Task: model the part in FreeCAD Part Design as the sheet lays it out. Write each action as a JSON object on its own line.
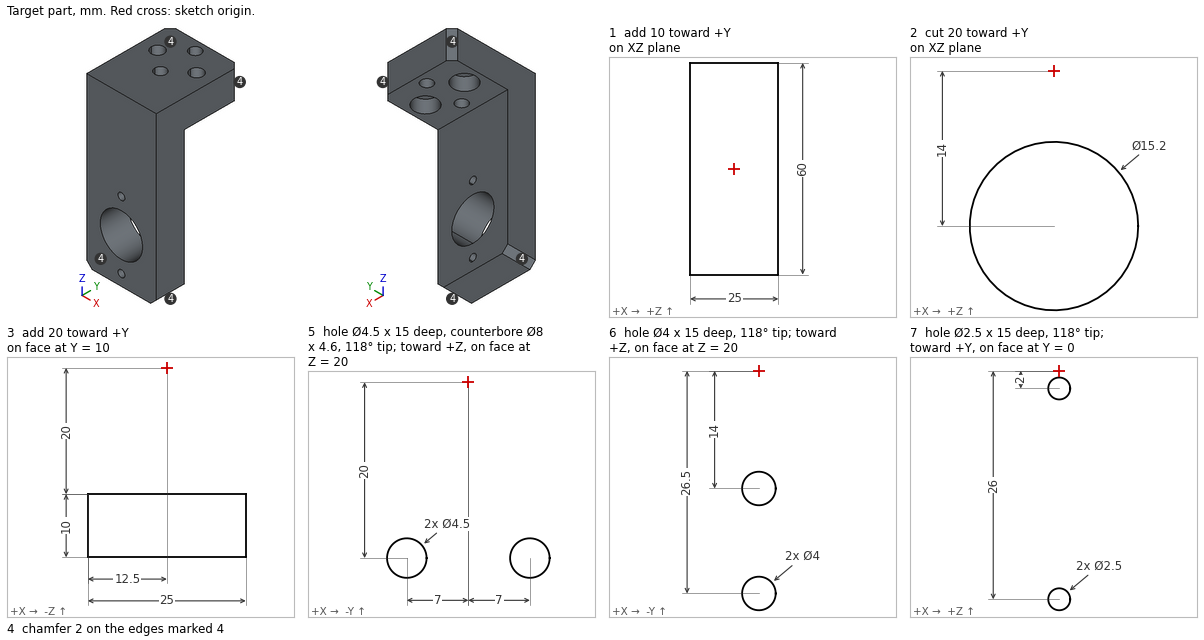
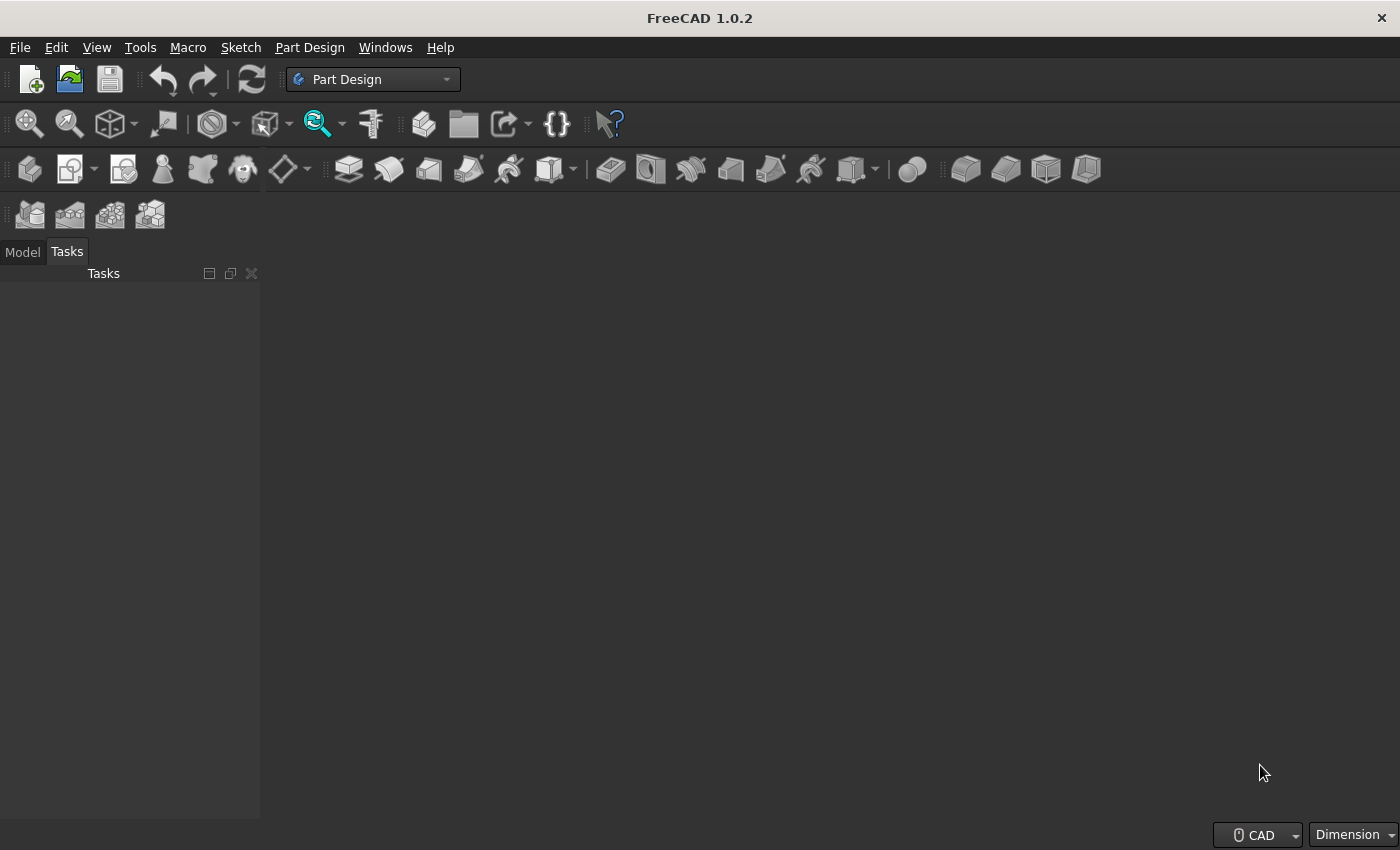
{"action": "left_click", "coordinate": [30, 80]}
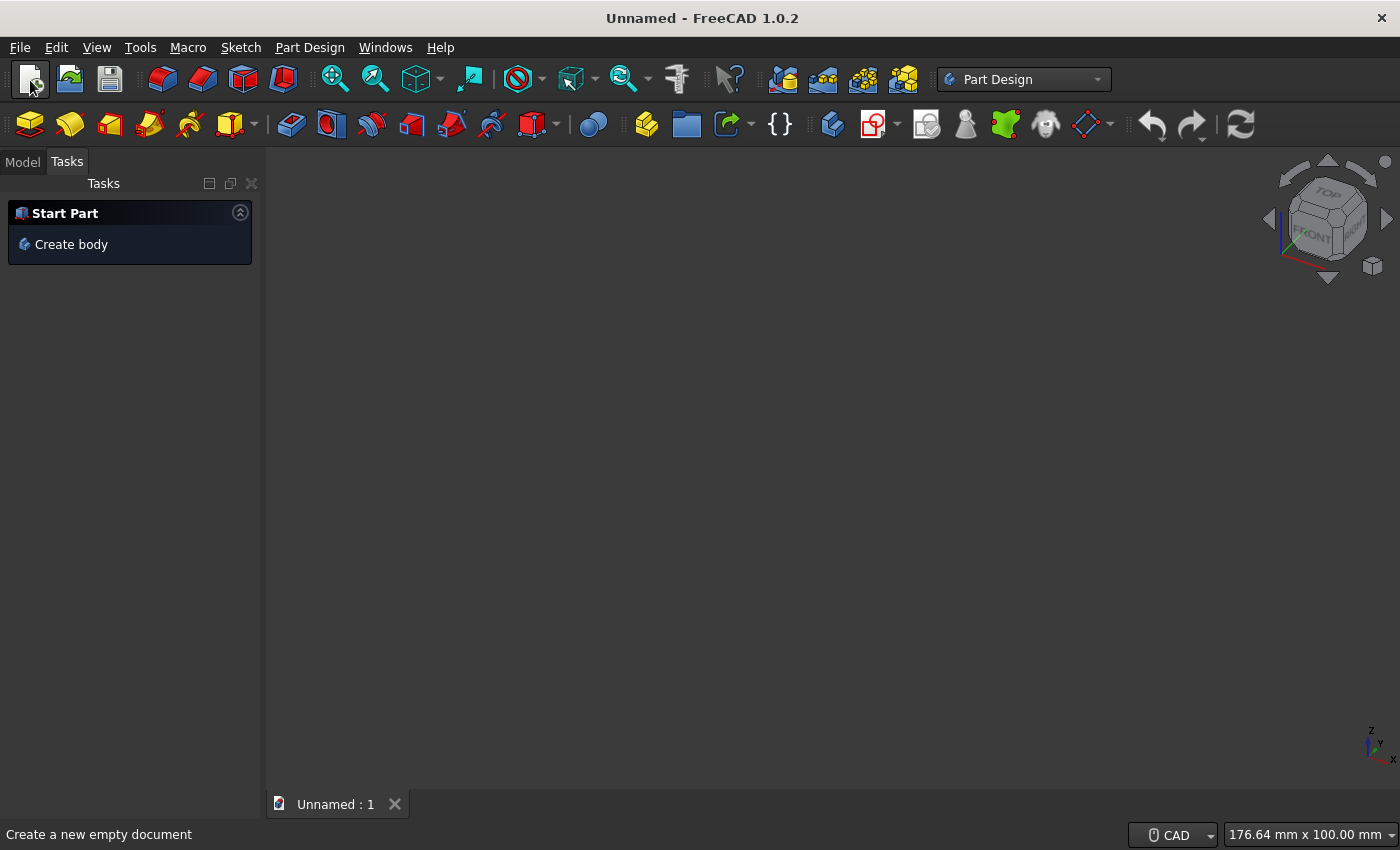
{"action": "left_click", "coordinate": [874, 124]}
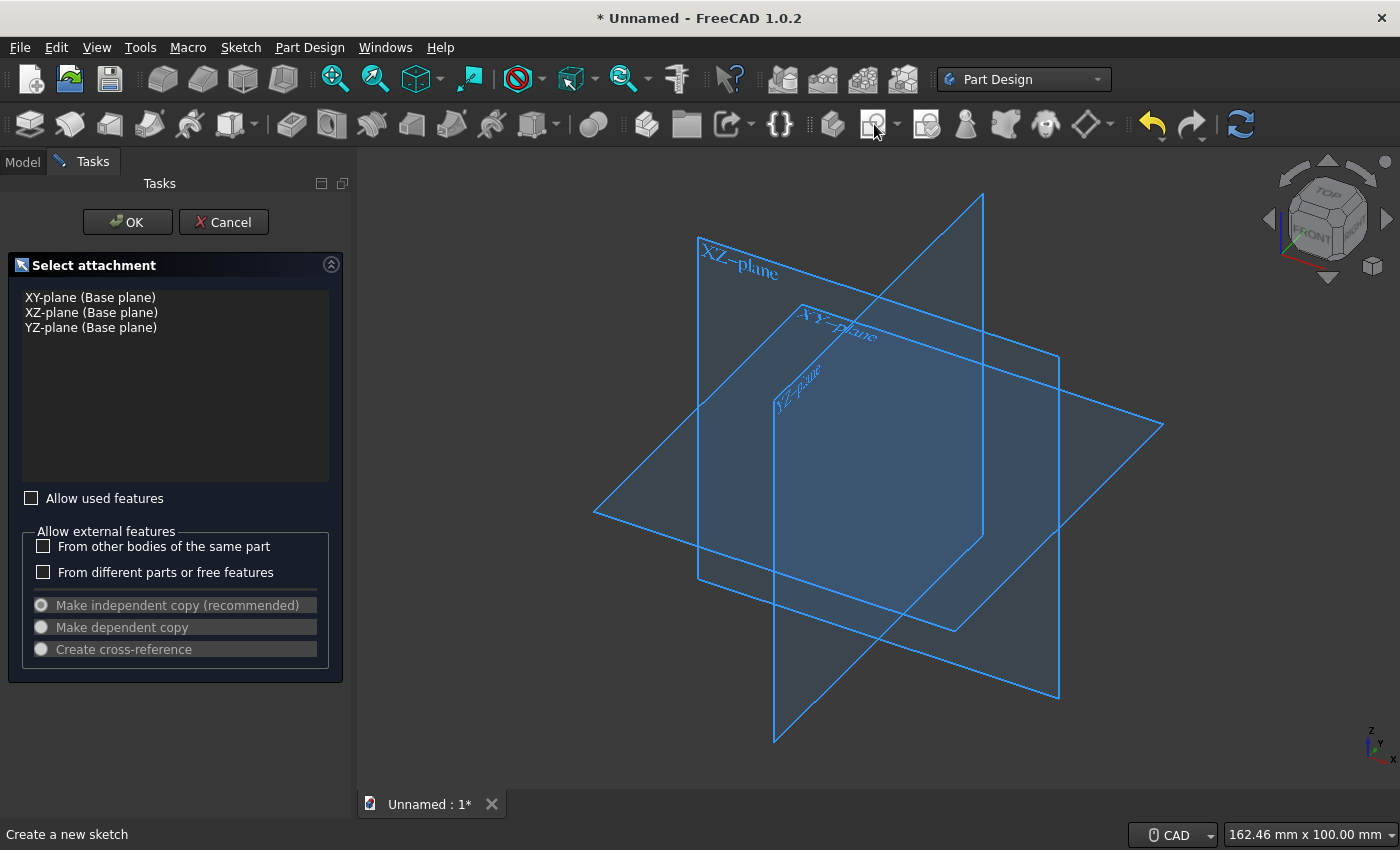
{"action": "left_click", "coordinate": [82, 312]}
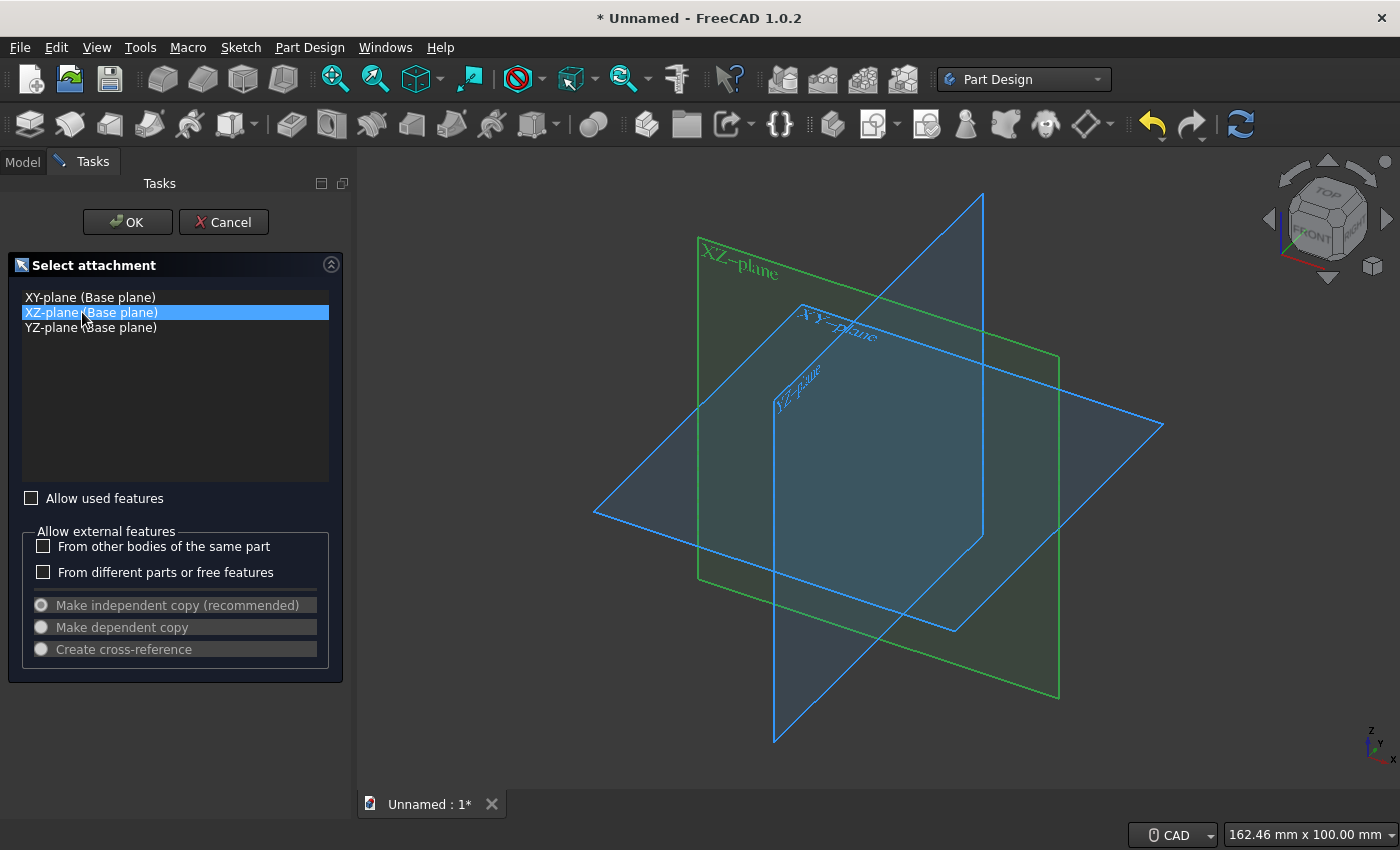
{"action": "left_click", "coordinate": [128, 222]}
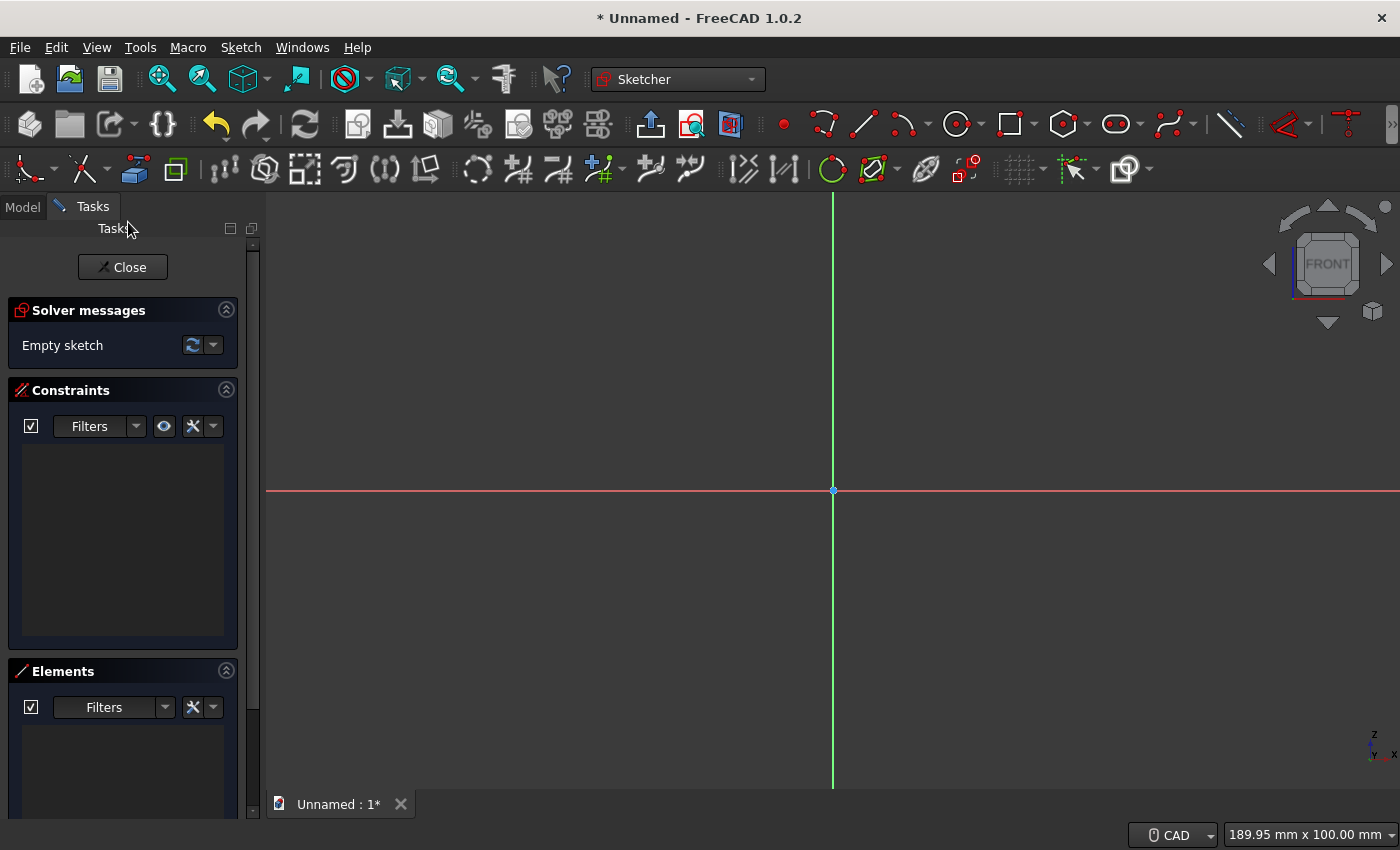
{"action": "key", "text": "g v"}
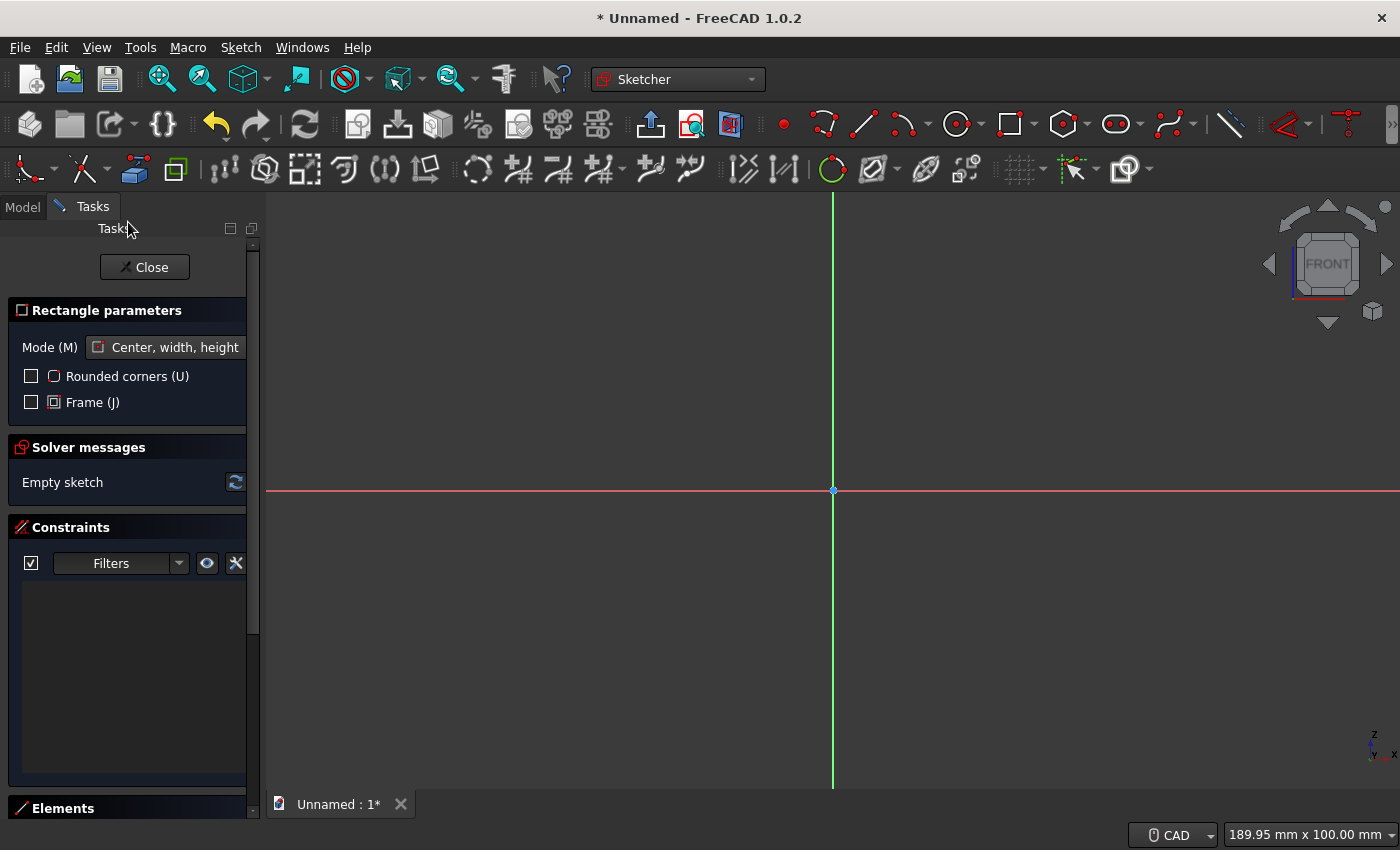
{"action": "left_click", "coordinate": [833, 490]}
{"action": "left_click", "coordinate": [908, 311]}
{"action": "key", "text": "Escape"}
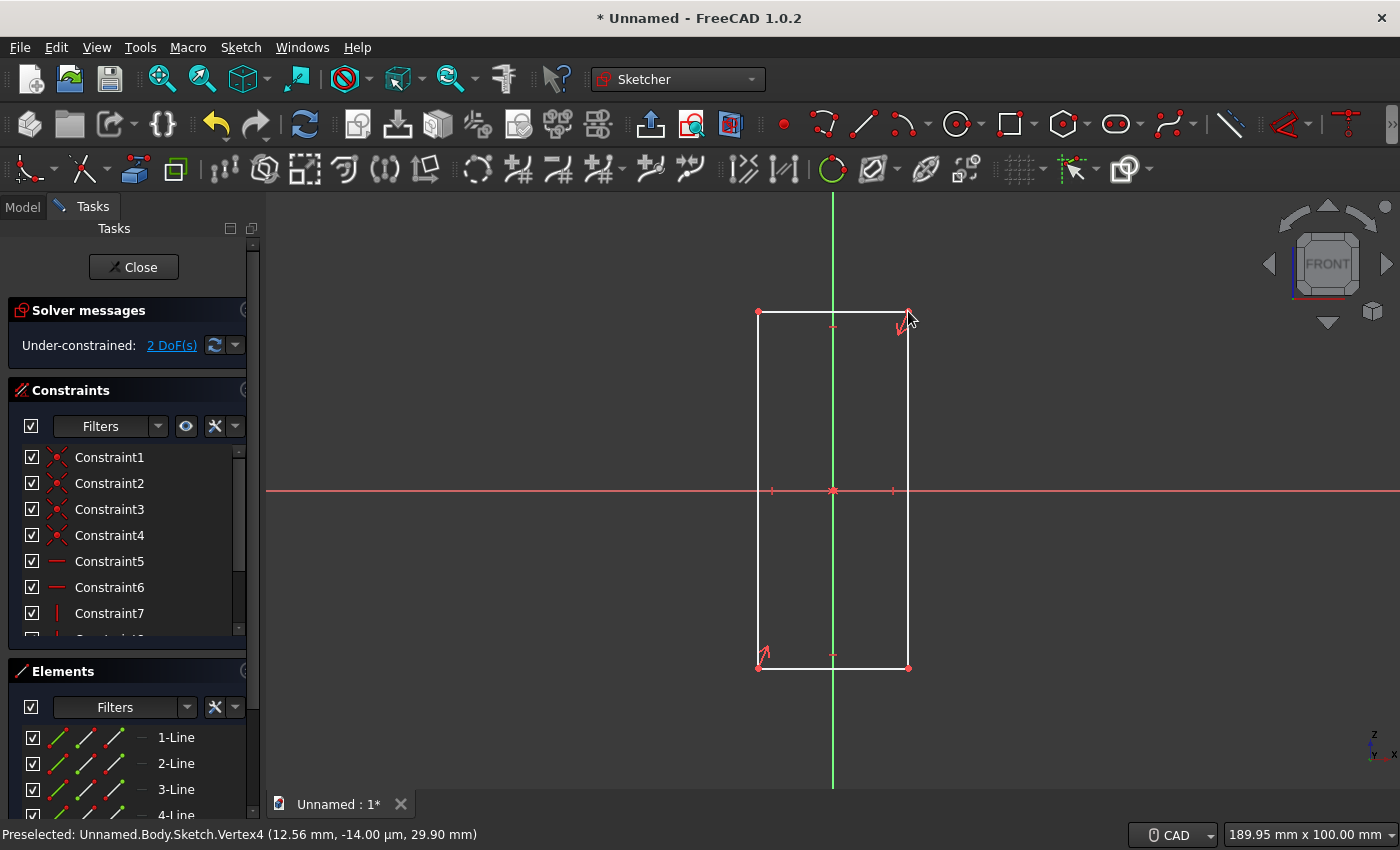
{"action": "left_click", "coordinate": [1284, 124]}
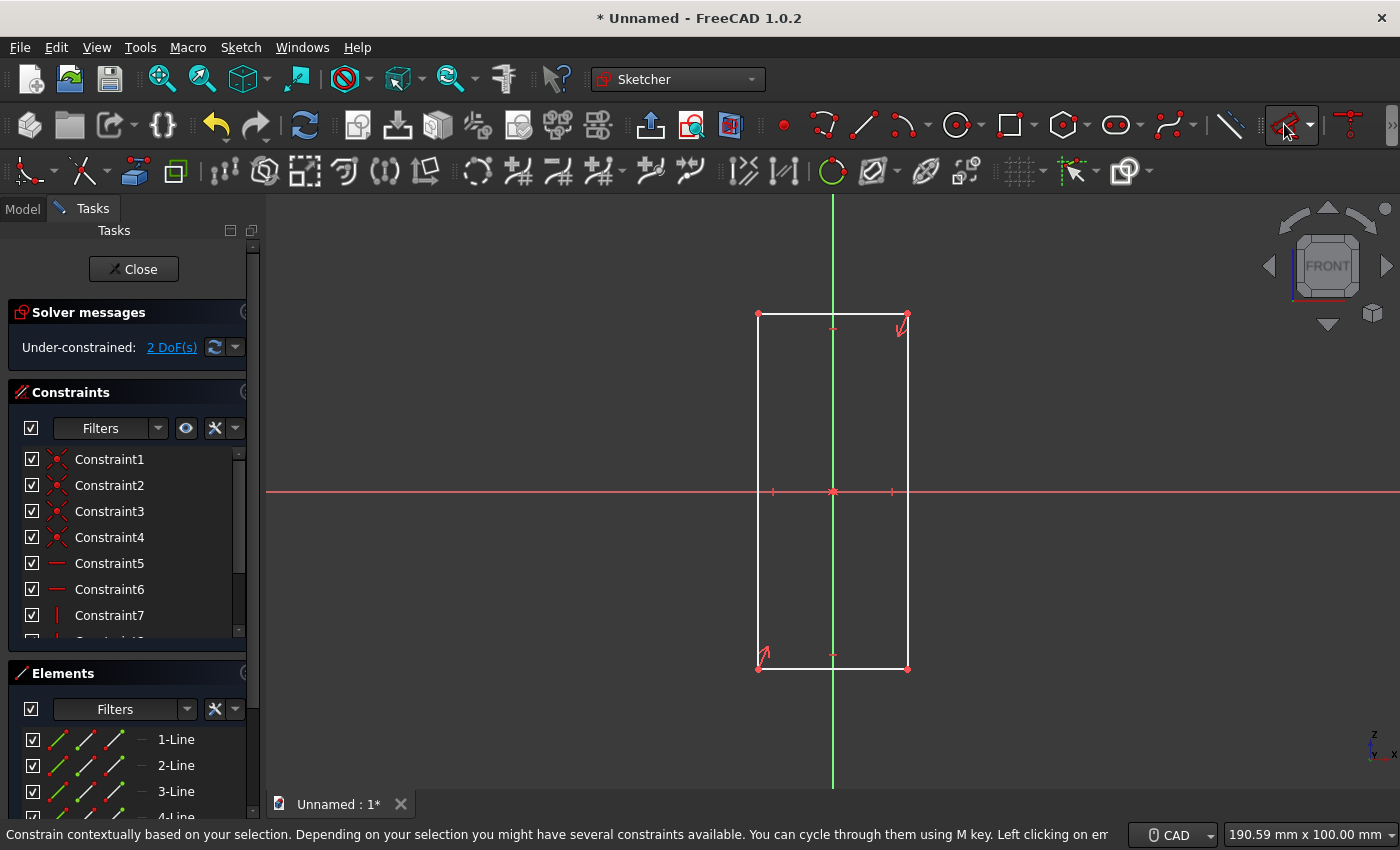
{"action": "left_click", "coordinate": [803, 669]}
{"action": "left_click", "coordinate": [799, 703]}